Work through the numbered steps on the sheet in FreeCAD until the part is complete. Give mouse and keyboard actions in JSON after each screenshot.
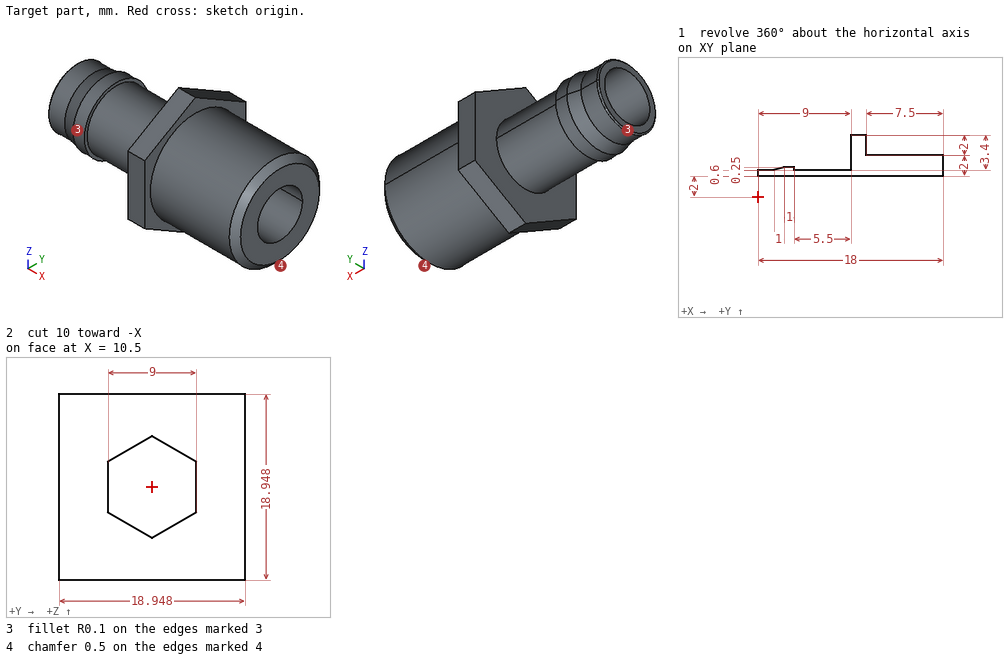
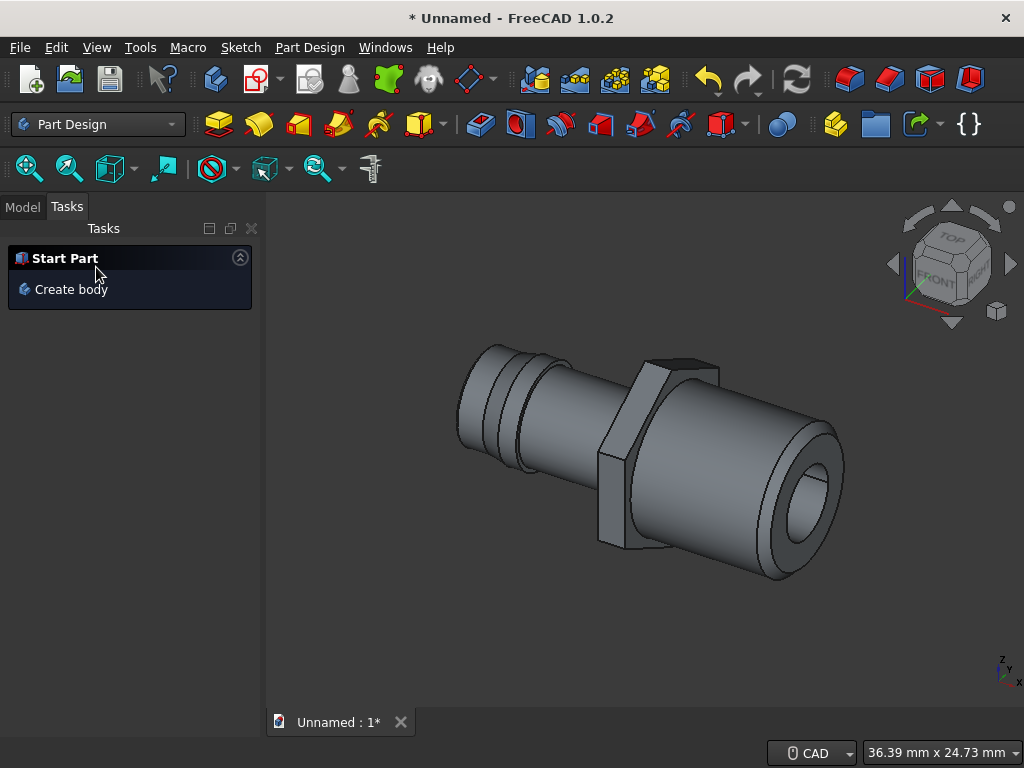
{"action": "key", "text": "0"}